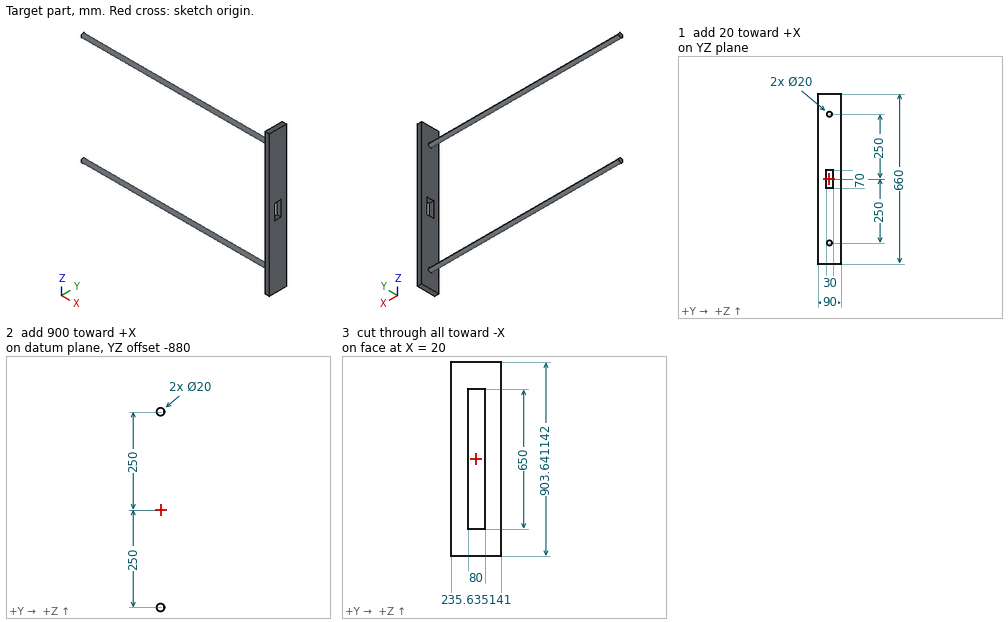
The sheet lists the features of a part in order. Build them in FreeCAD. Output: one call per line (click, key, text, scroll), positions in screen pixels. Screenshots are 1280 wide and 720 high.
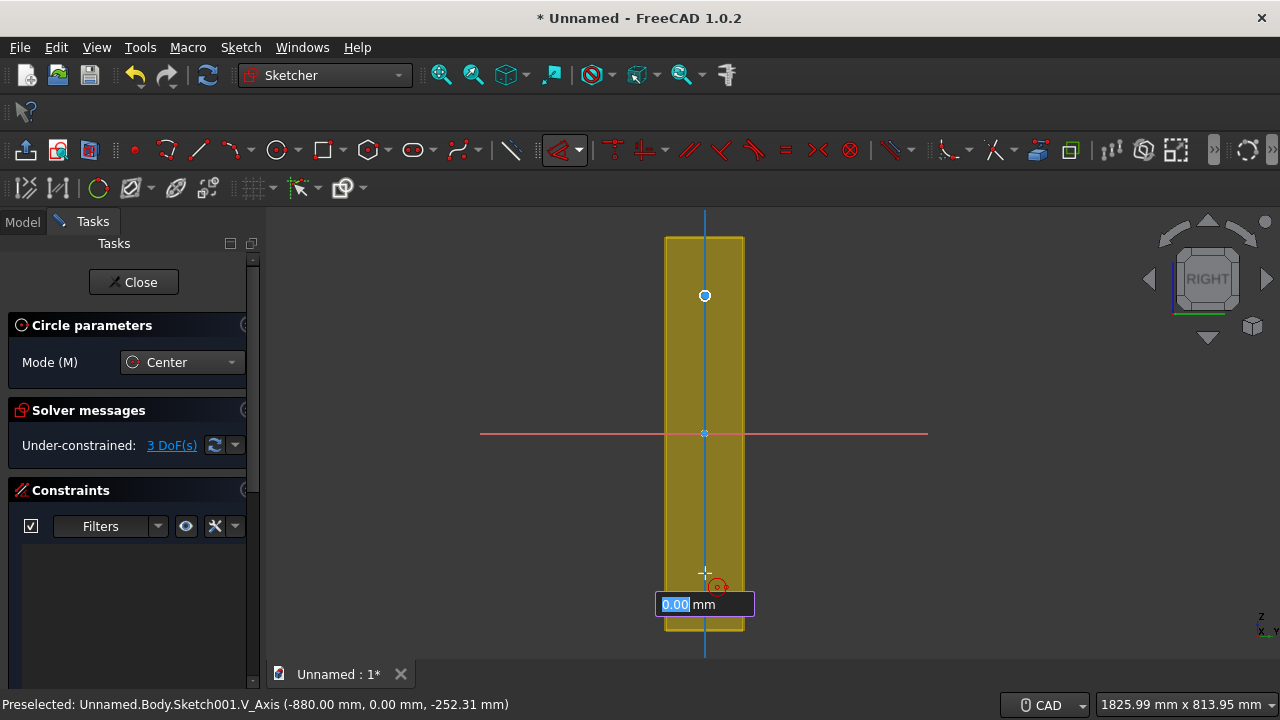
scroll(710, 571, up, 6)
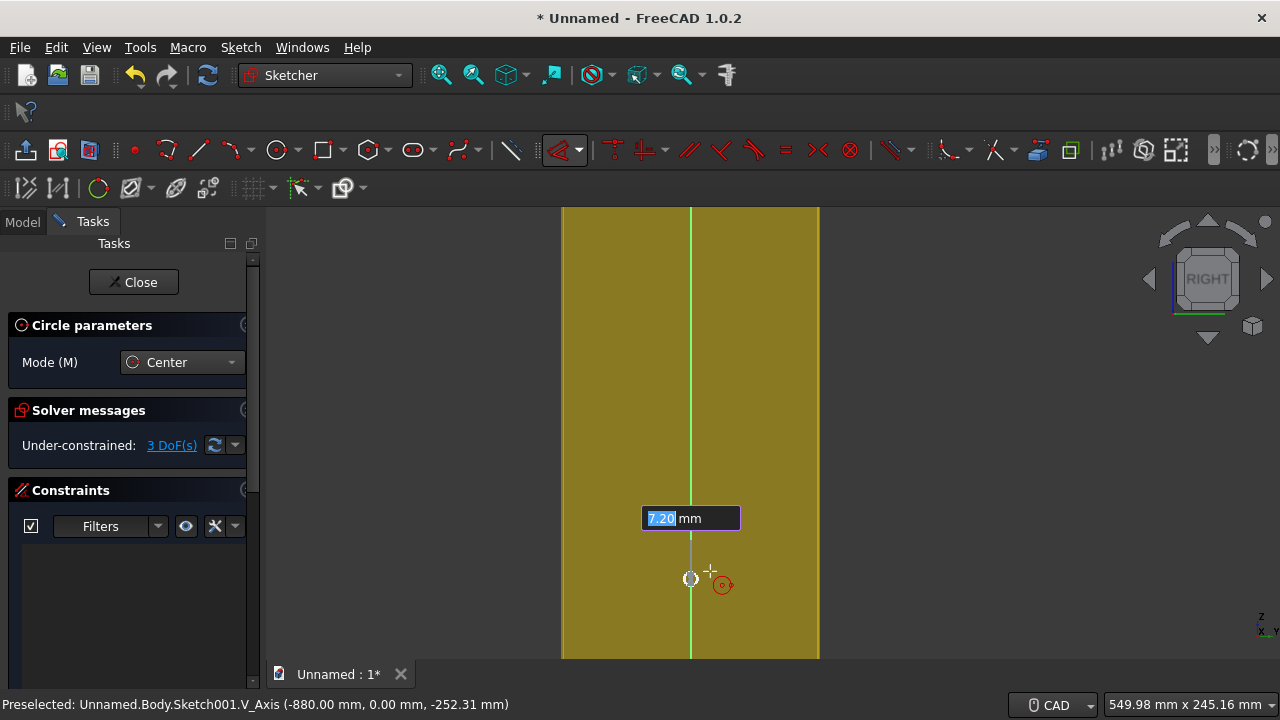
click(708, 569)
key(Escape)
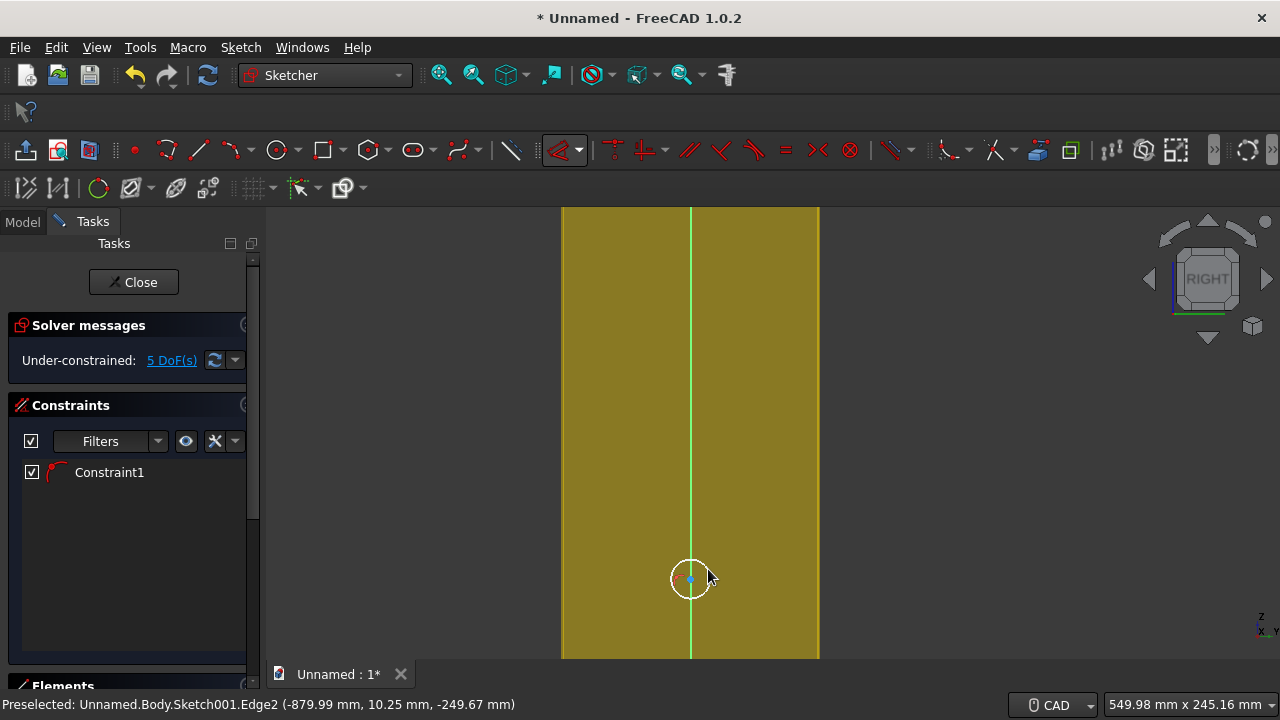
scroll(710, 571, down, 6)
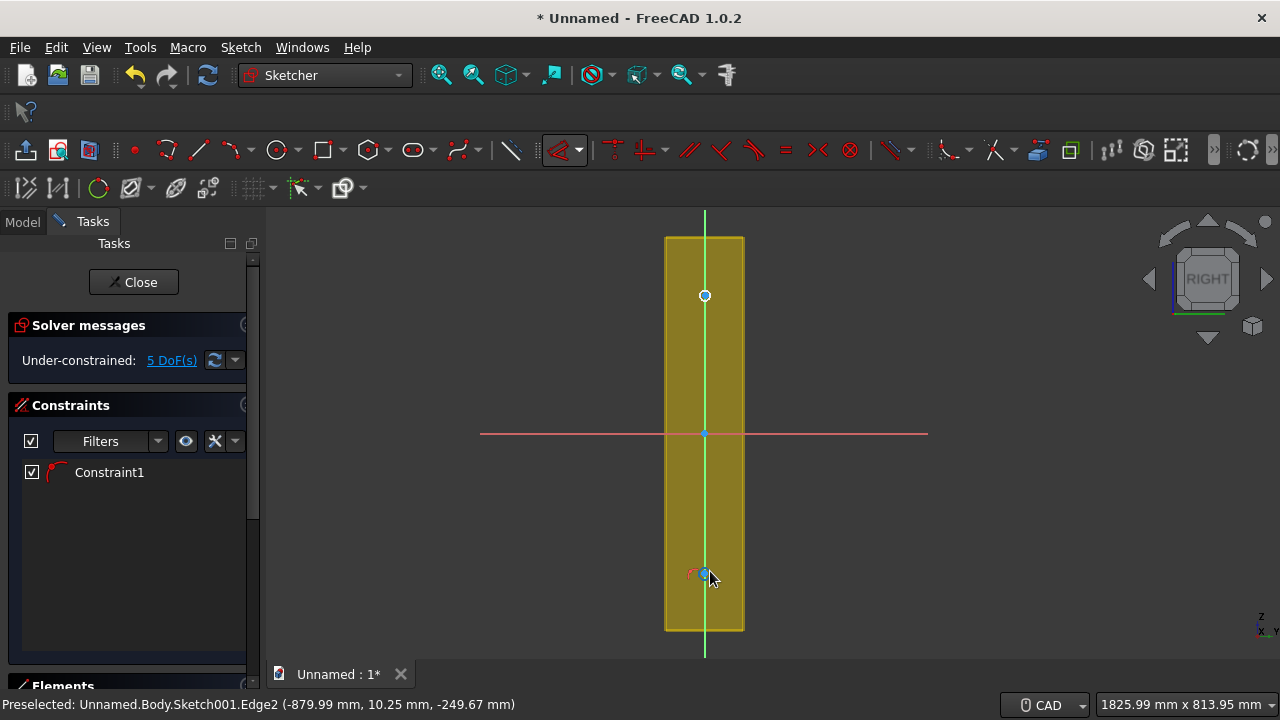
scroll(709, 292, up, 6)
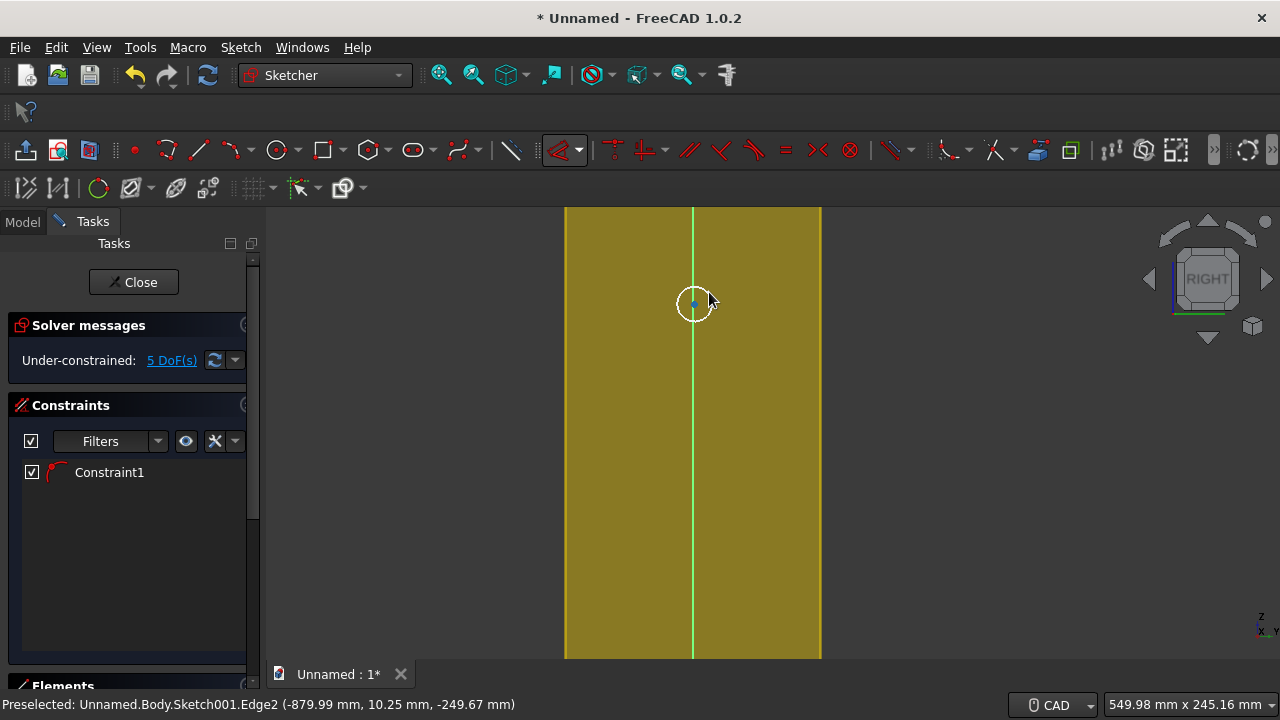
click(707, 292)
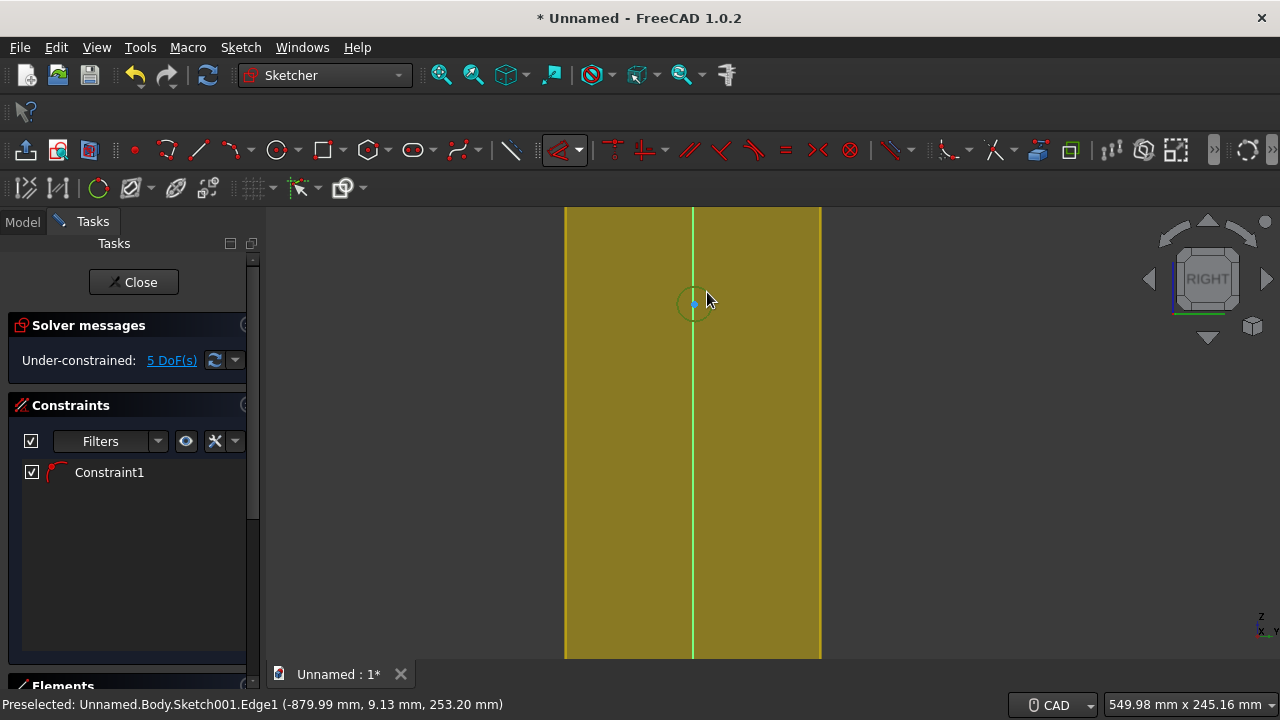
scroll(709, 291, down, 6)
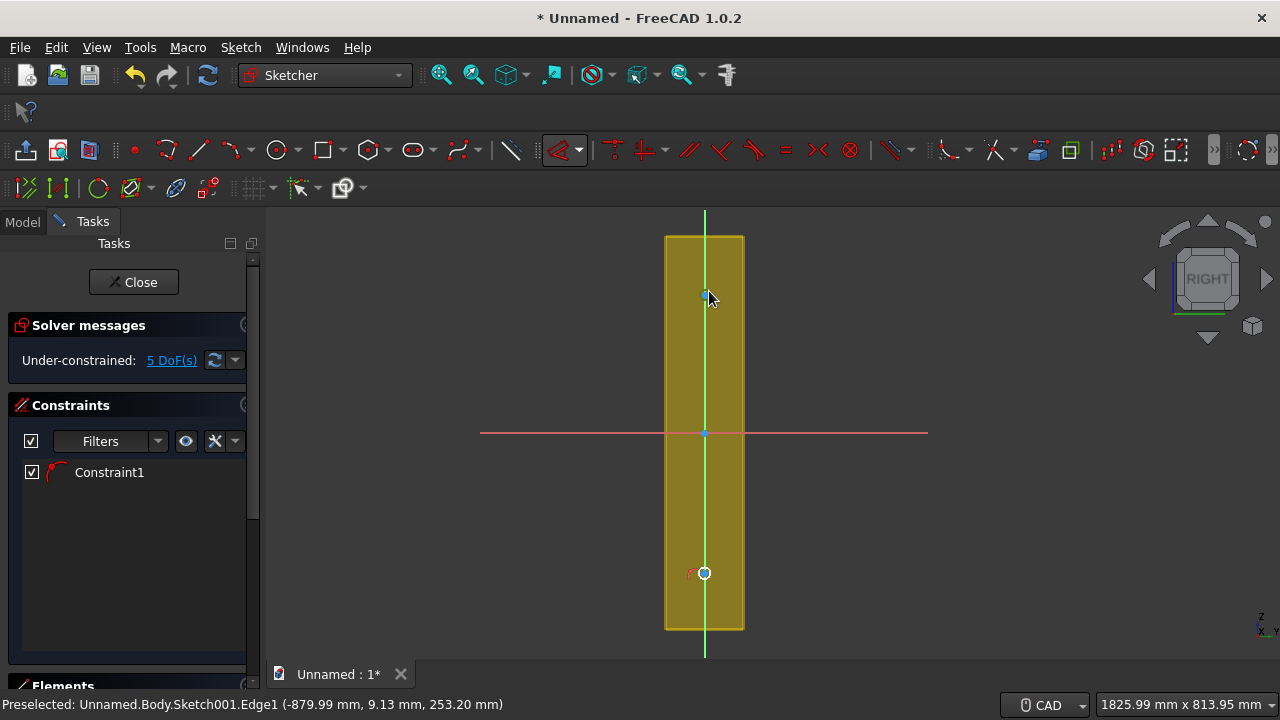
scroll(709, 569, up, 7)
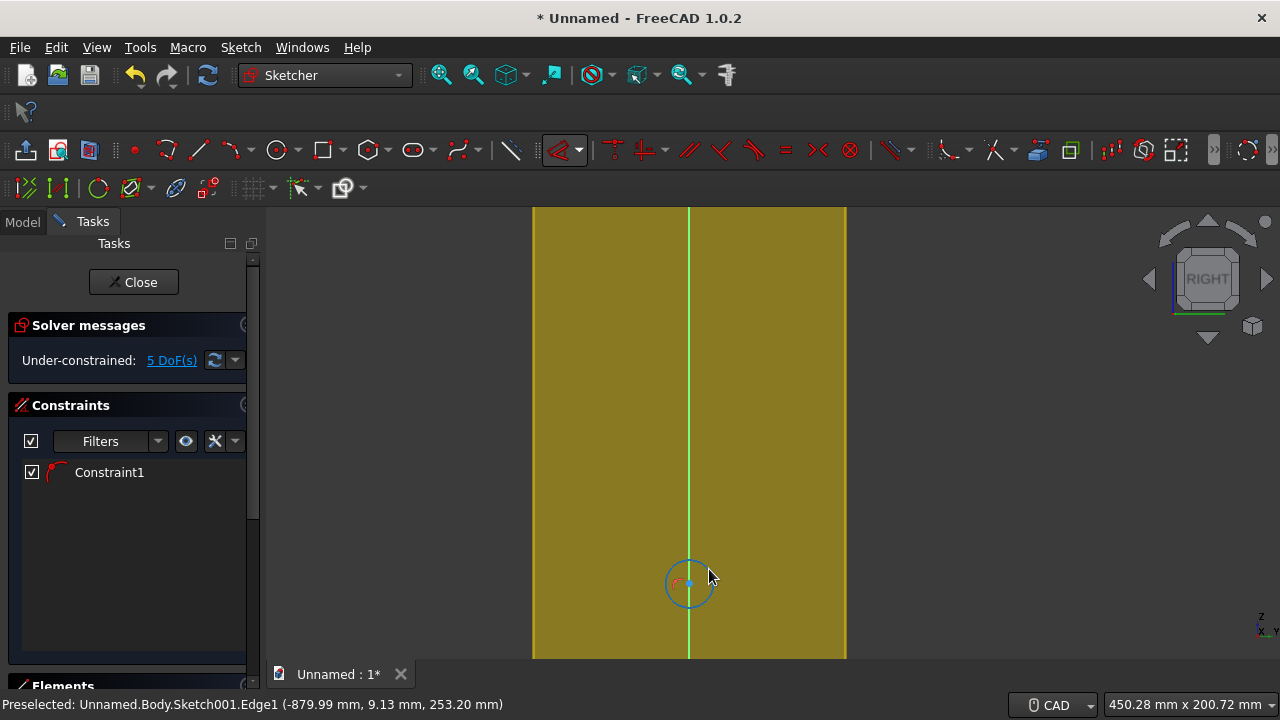
click(706, 567)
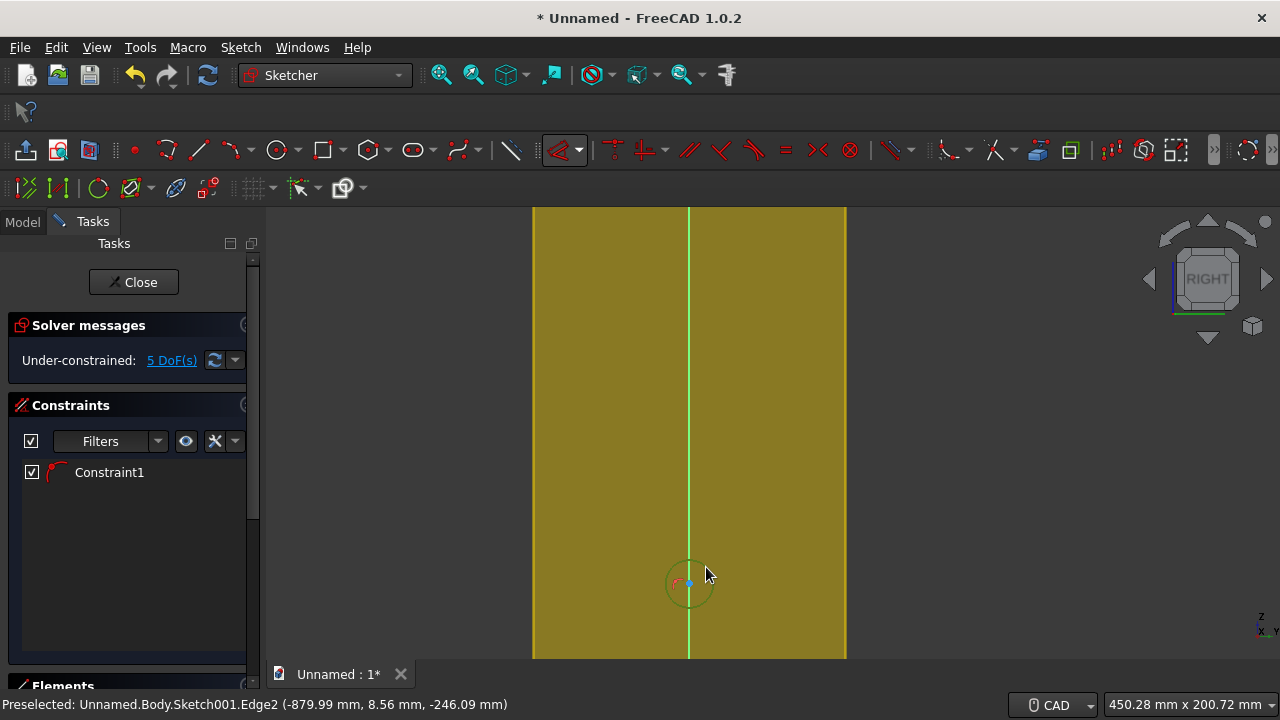
key(e)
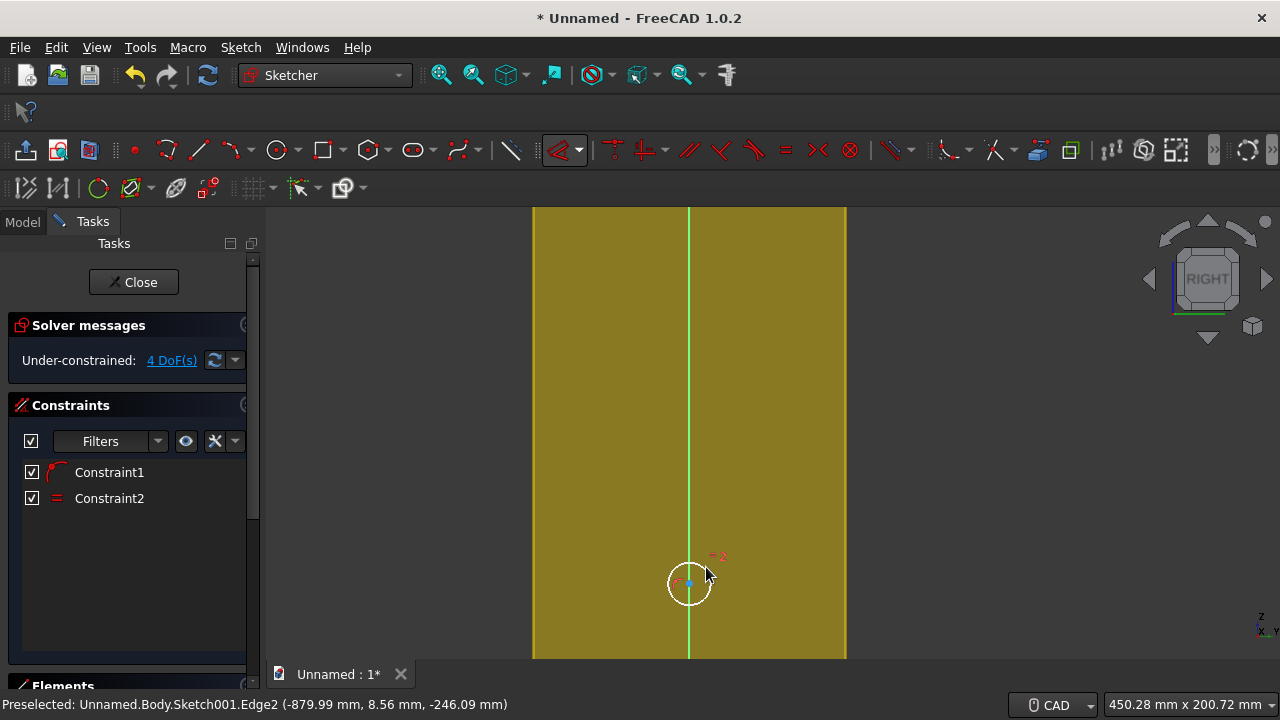
scroll(709, 570, down, 7)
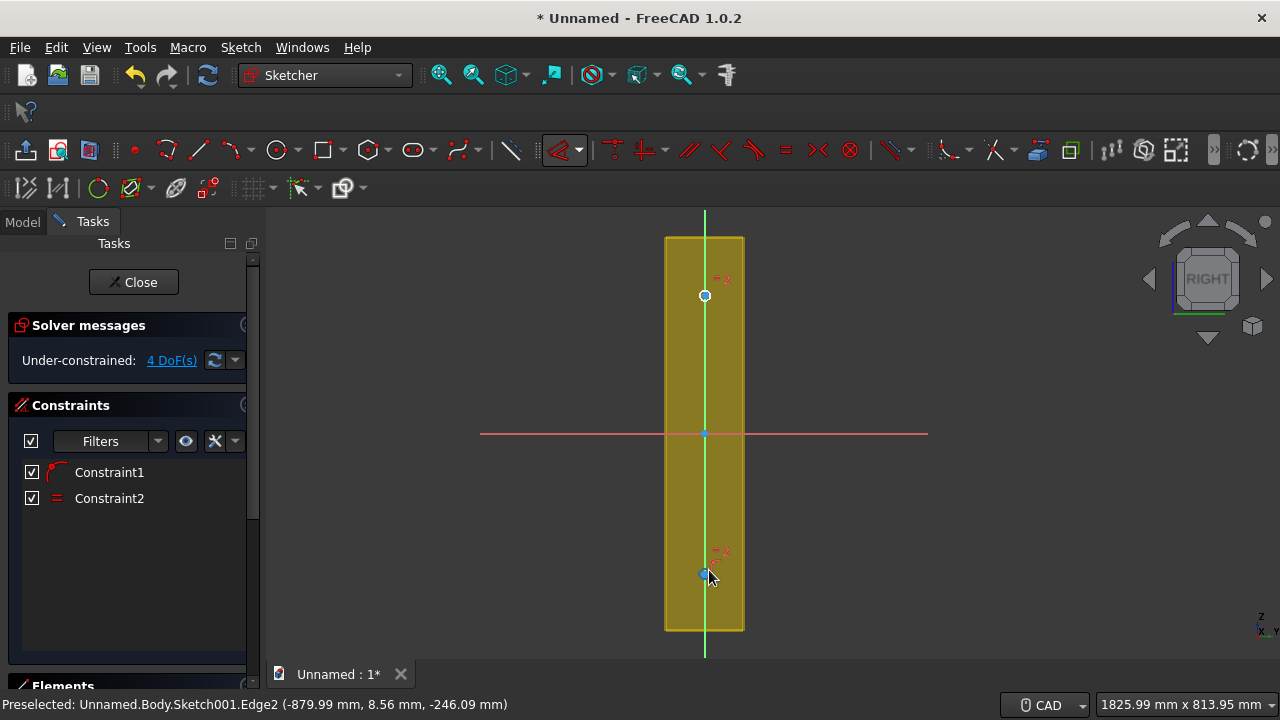
click(705, 296)